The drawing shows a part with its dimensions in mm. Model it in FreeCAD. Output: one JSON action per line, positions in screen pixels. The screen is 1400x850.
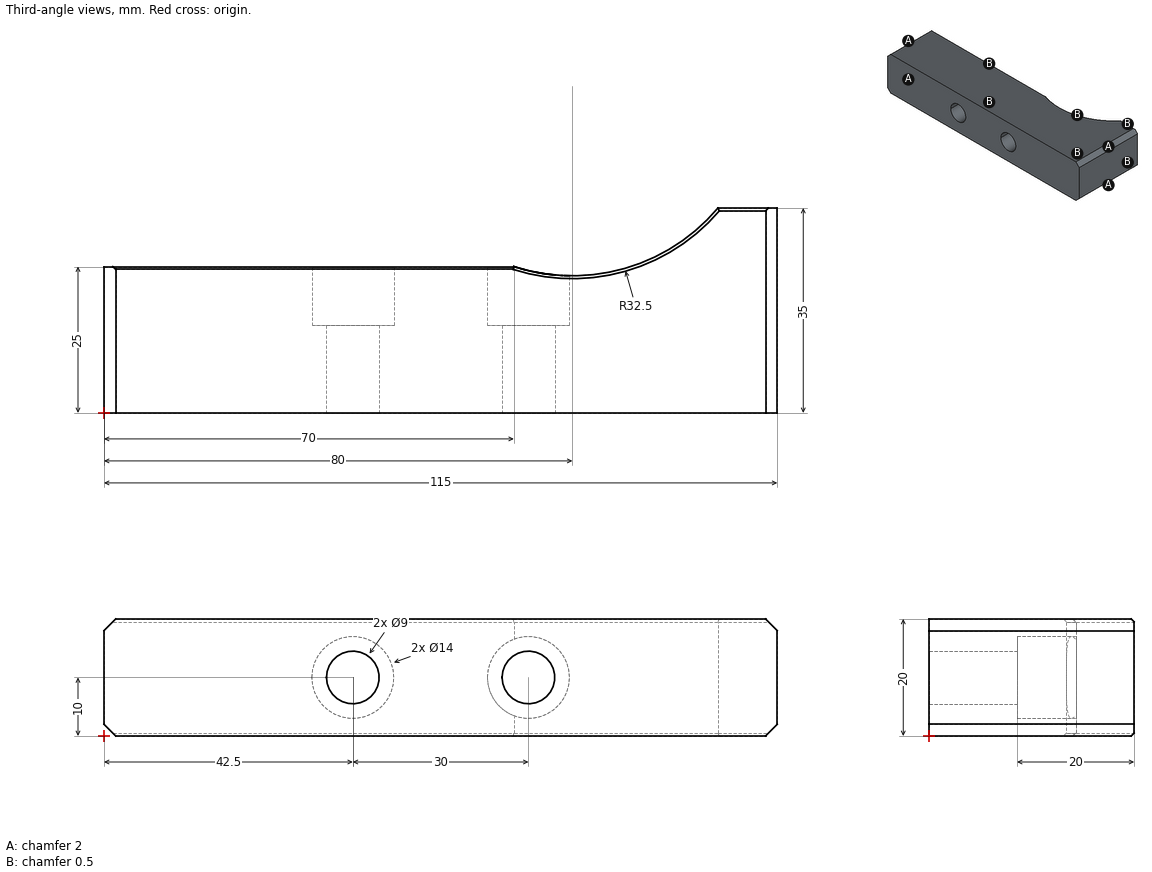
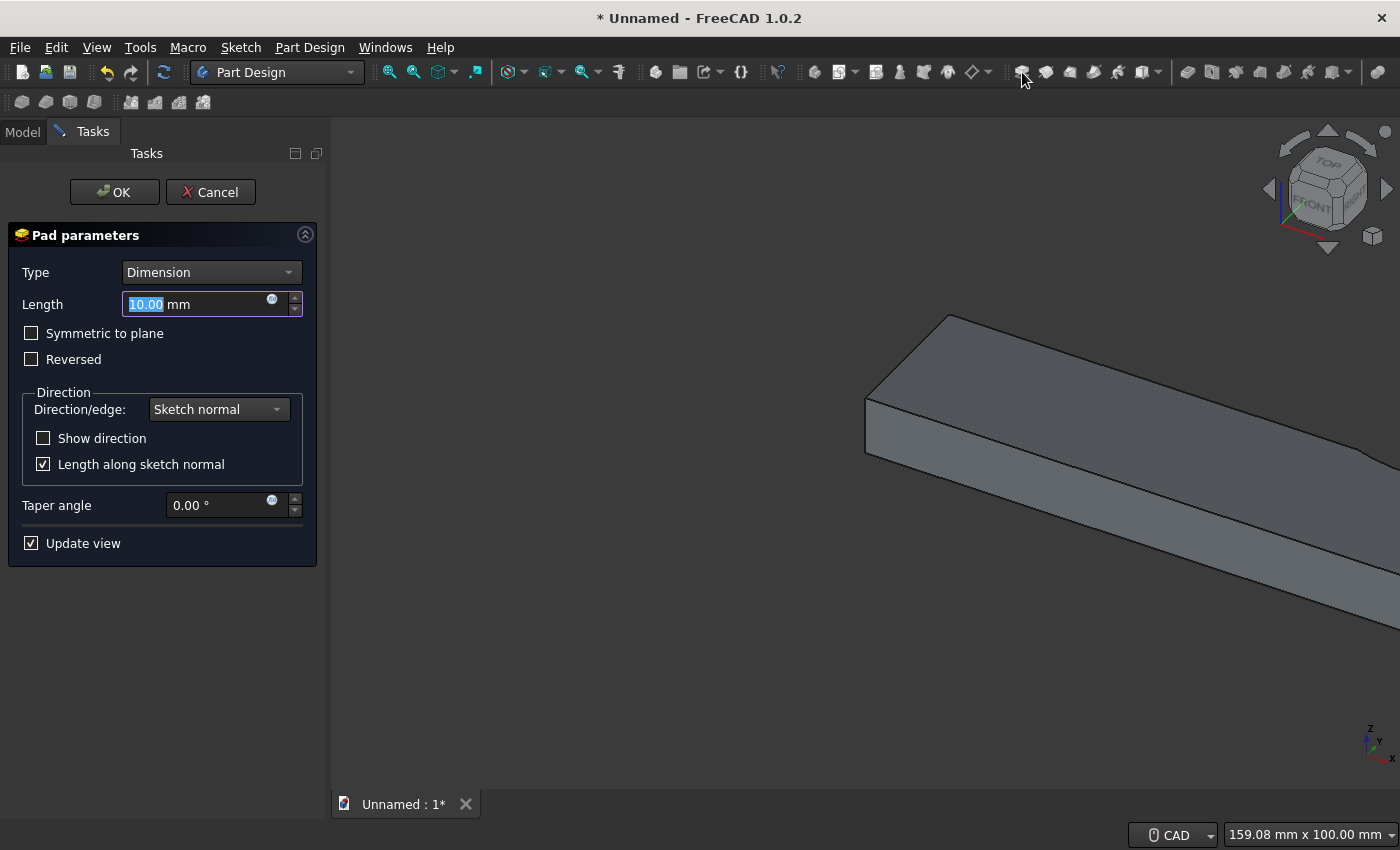
{"action": "type", "text": "20"}
{"action": "key", "text": "Tab"}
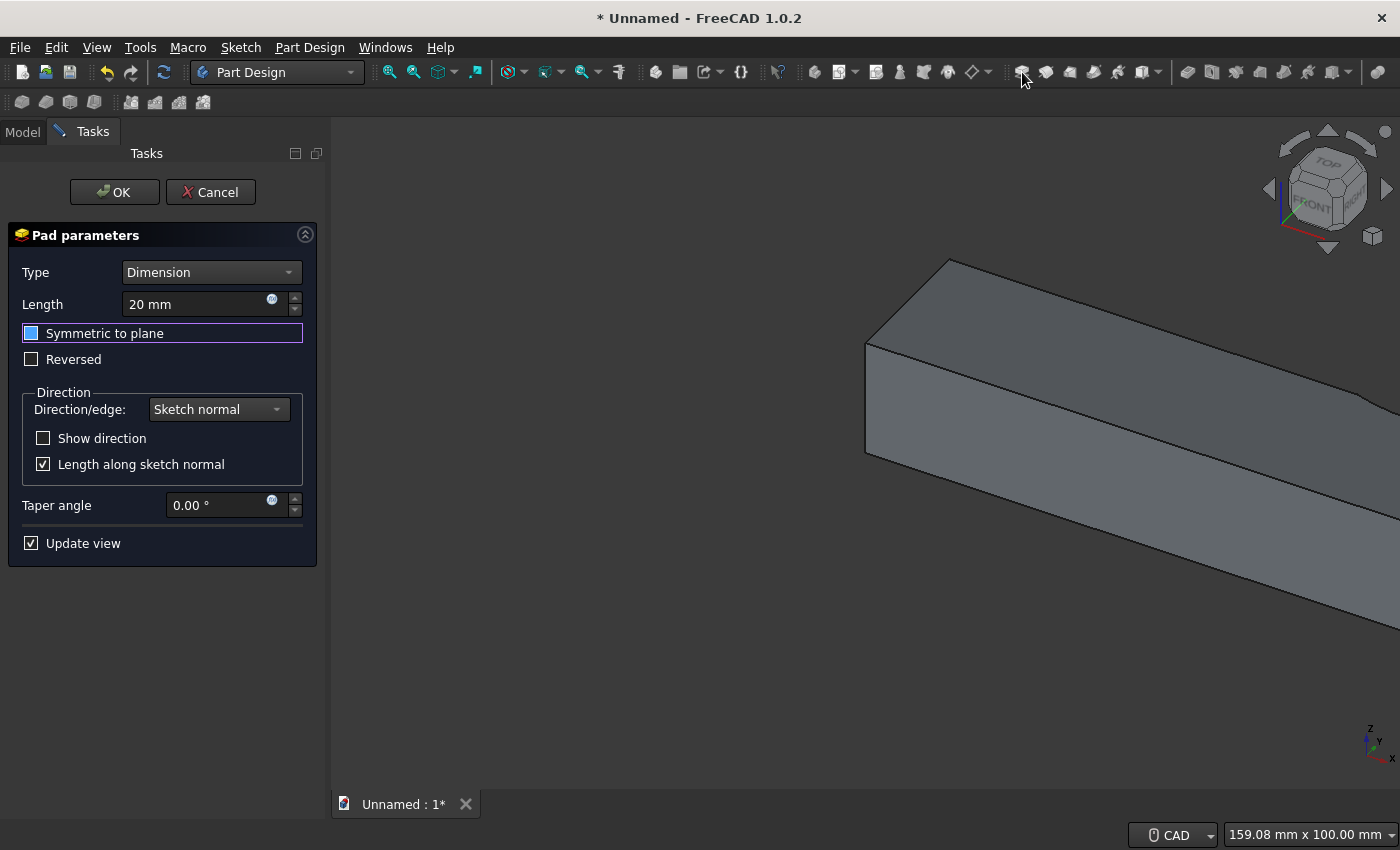
{"action": "left_click", "coordinate": [115, 192]}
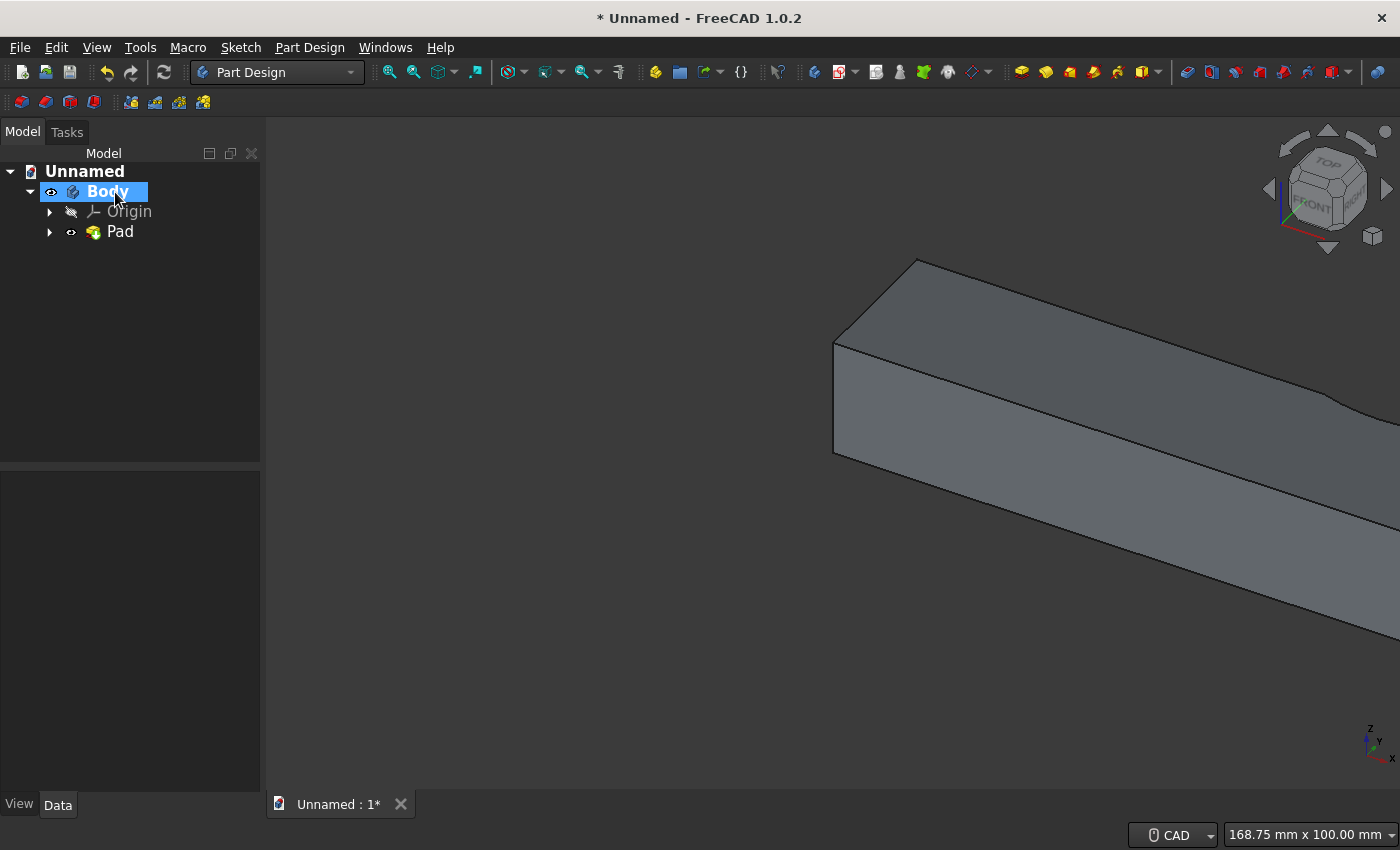
{"action": "left_click", "coordinate": [390, 72]}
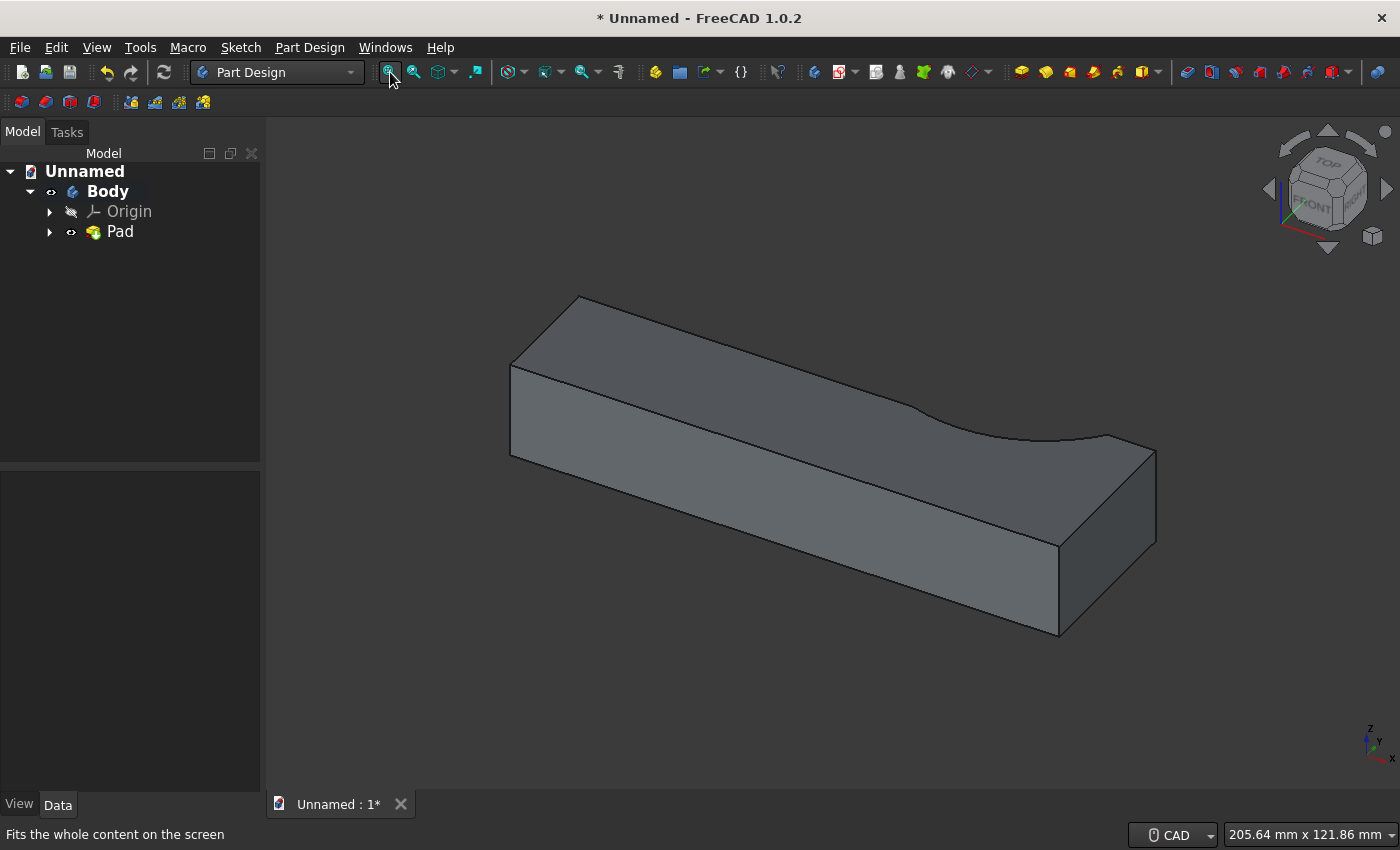
{"action": "key", "text": "4"}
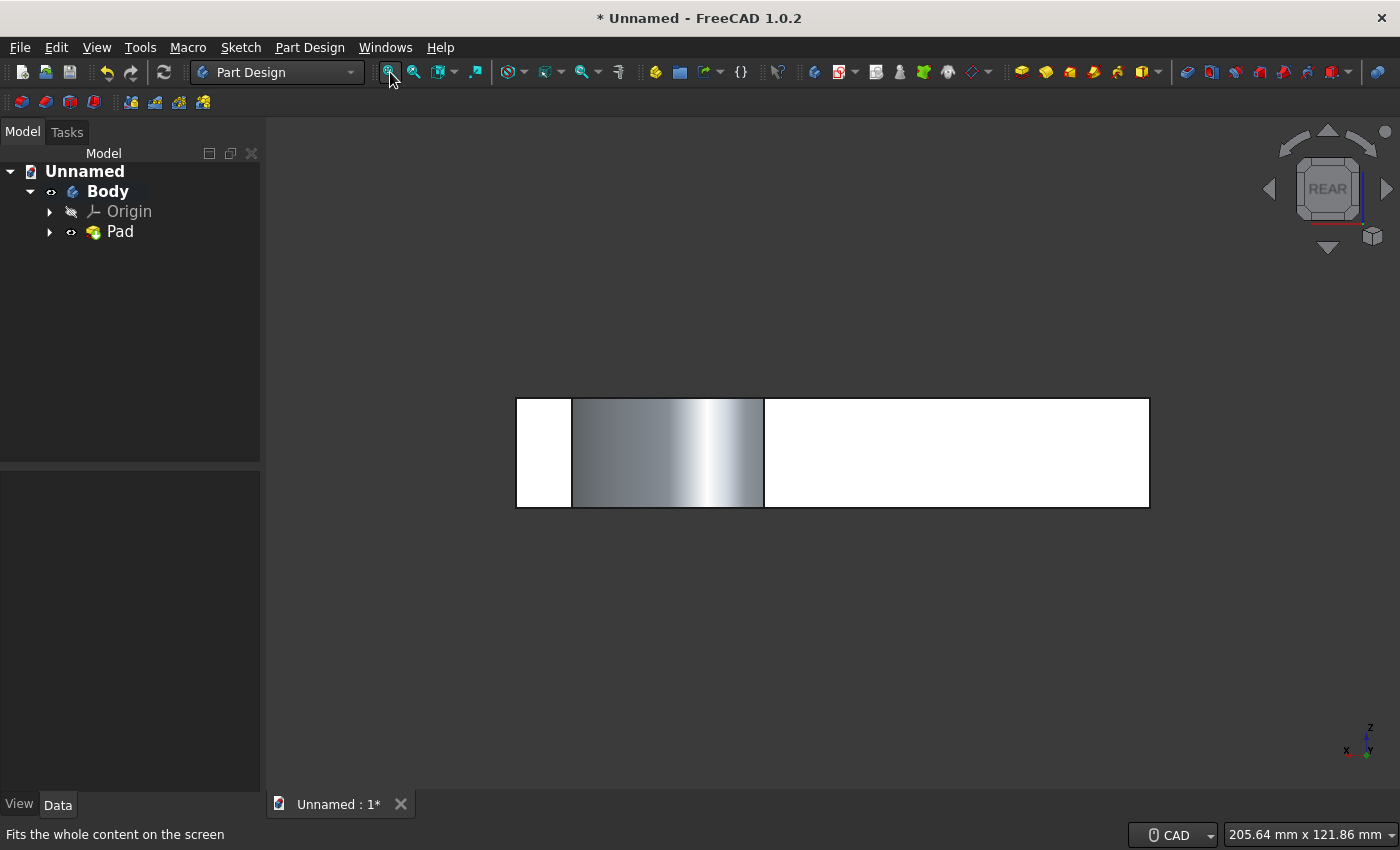
{"action": "left_click", "coordinate": [544, 436]}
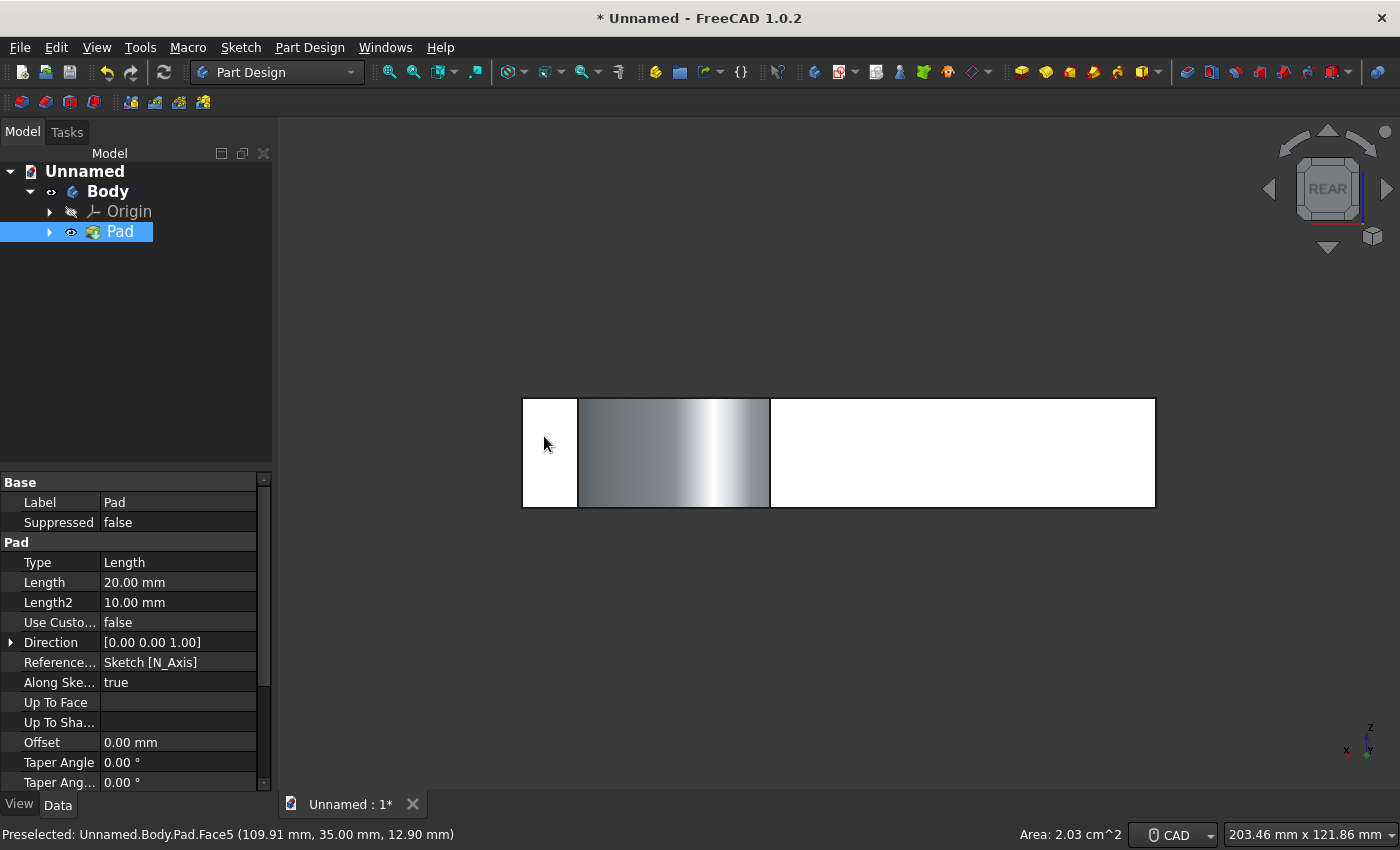
{"action": "left_click", "coordinate": [840, 72]}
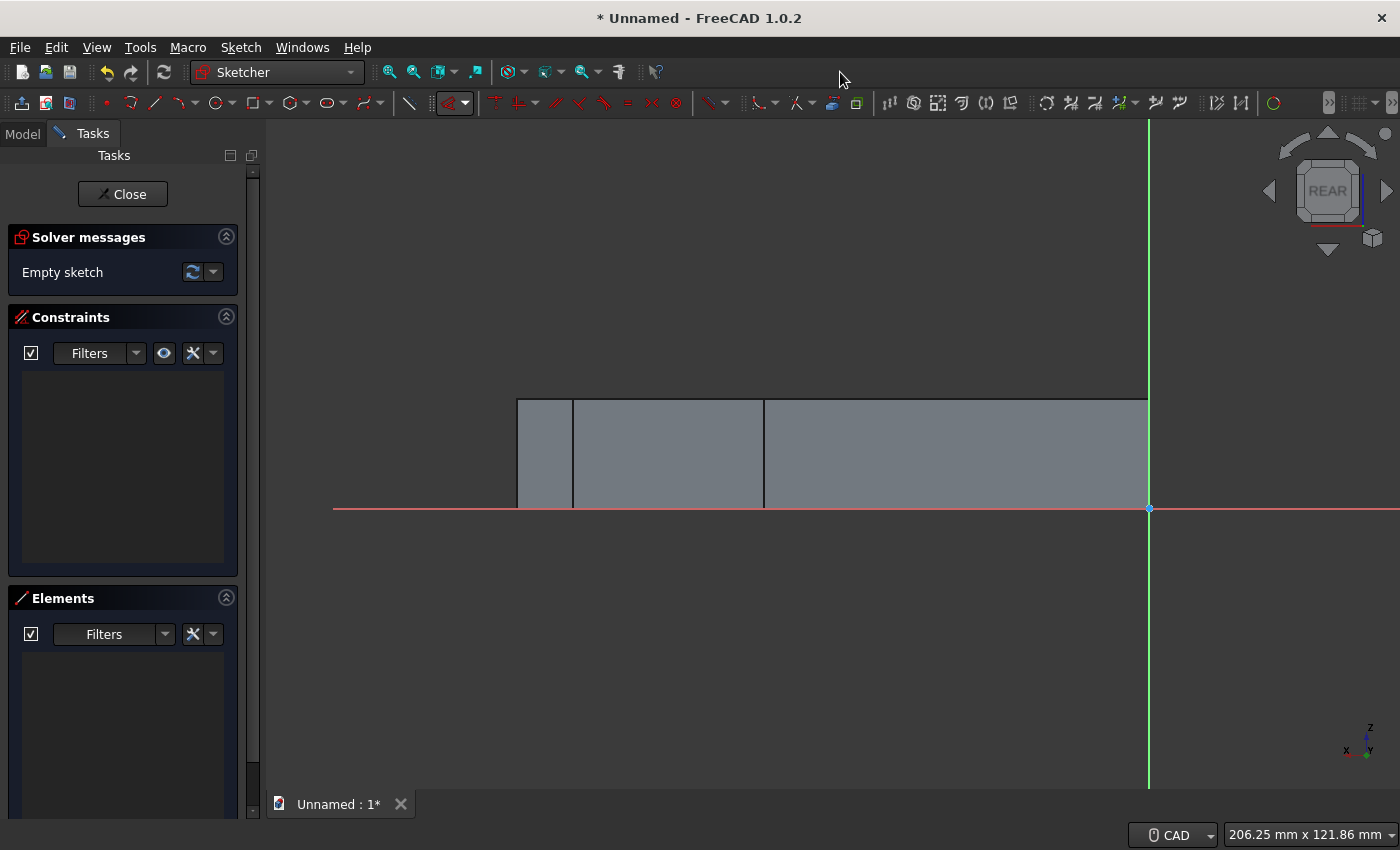
{"action": "scroll", "coordinate": [1235, 479], "scroll_direction": "up", "scroll_amount": 2}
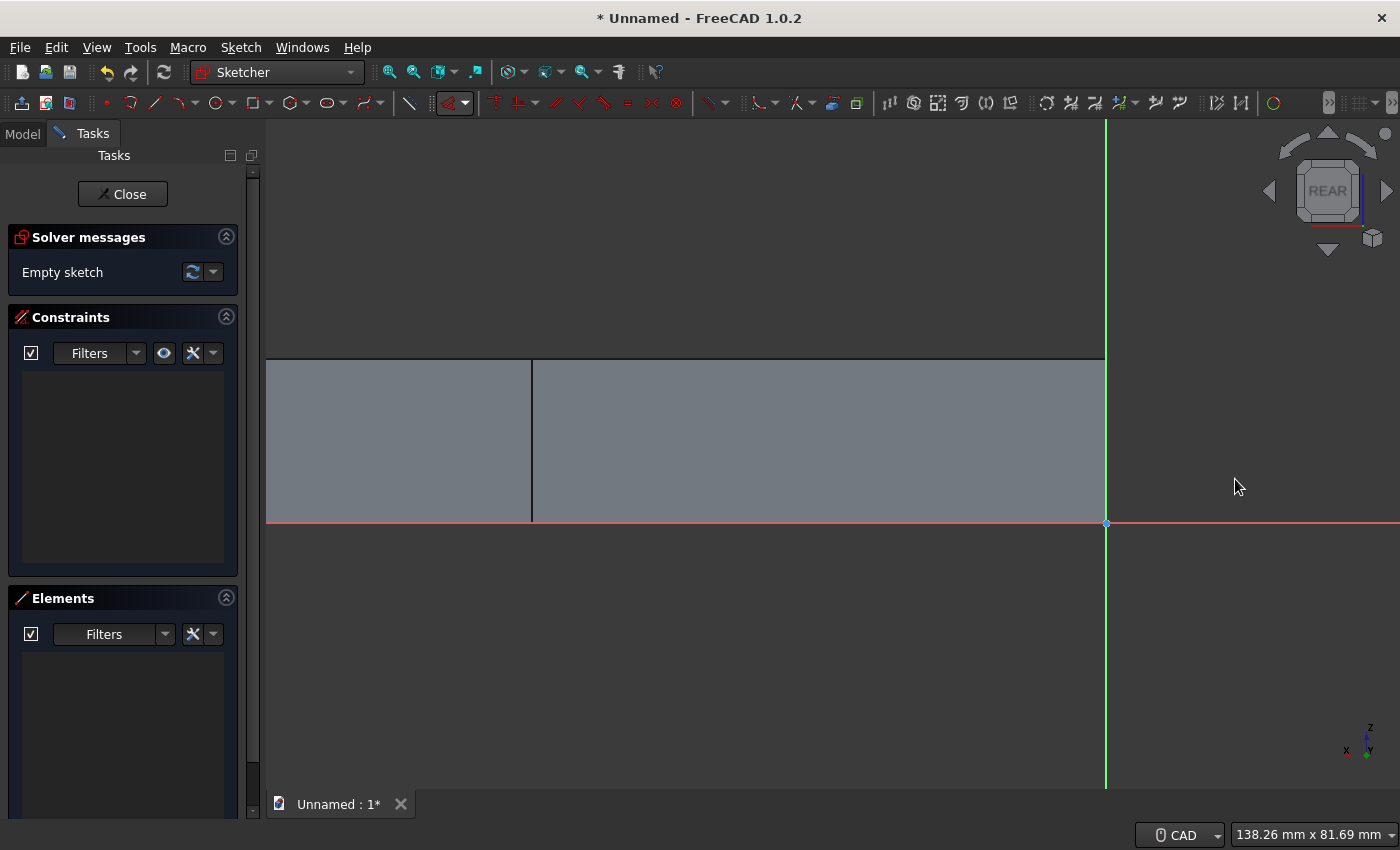
{"action": "left_click", "coordinate": [216, 104]}